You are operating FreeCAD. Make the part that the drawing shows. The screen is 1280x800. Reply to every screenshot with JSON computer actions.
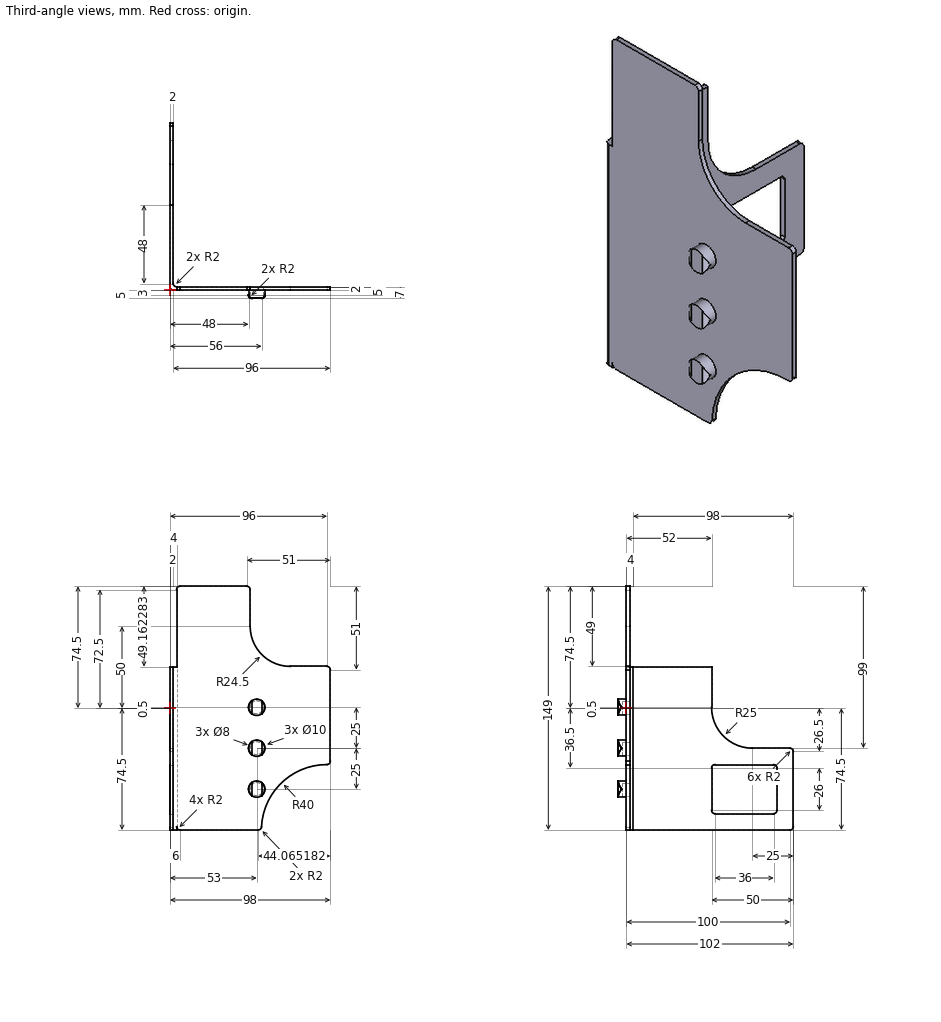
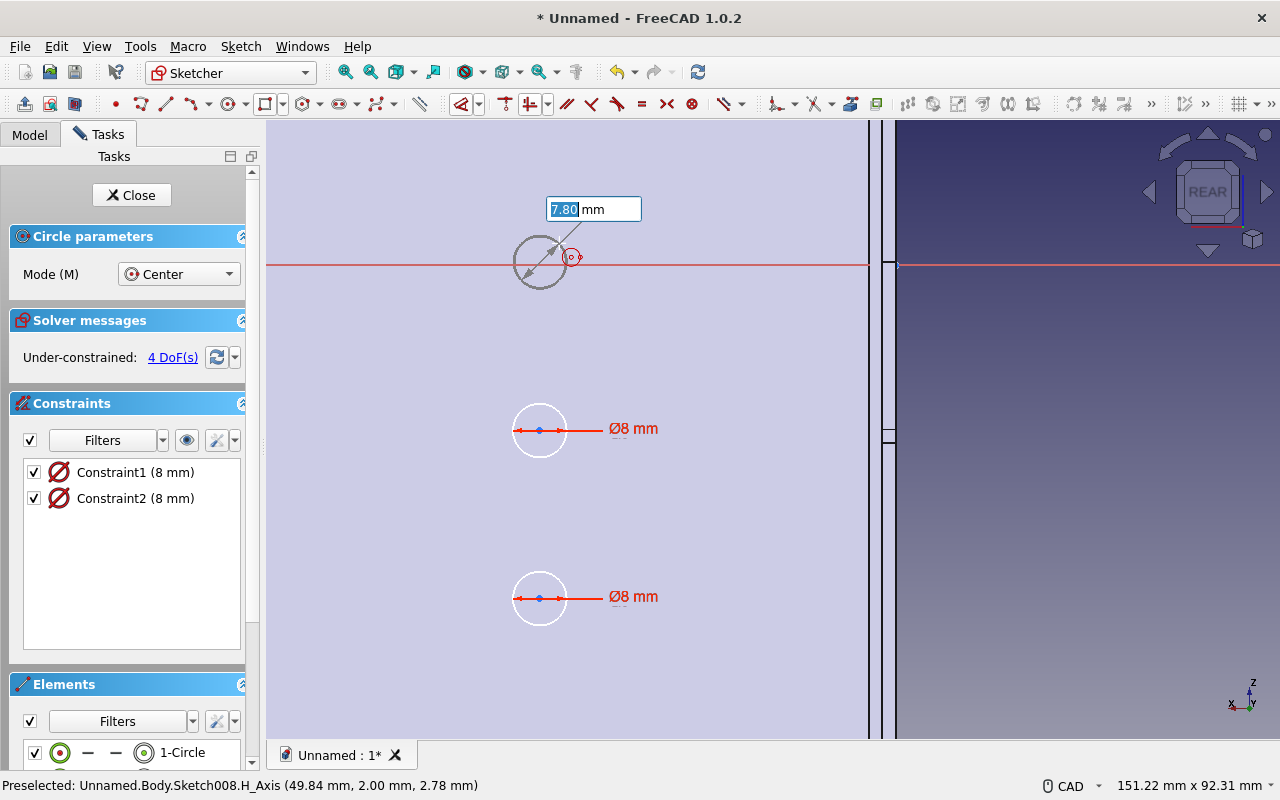
{"action": "type", "text": "8"}
{"action": "key", "text": "Return"}
{"action": "key", "text": "Escape"}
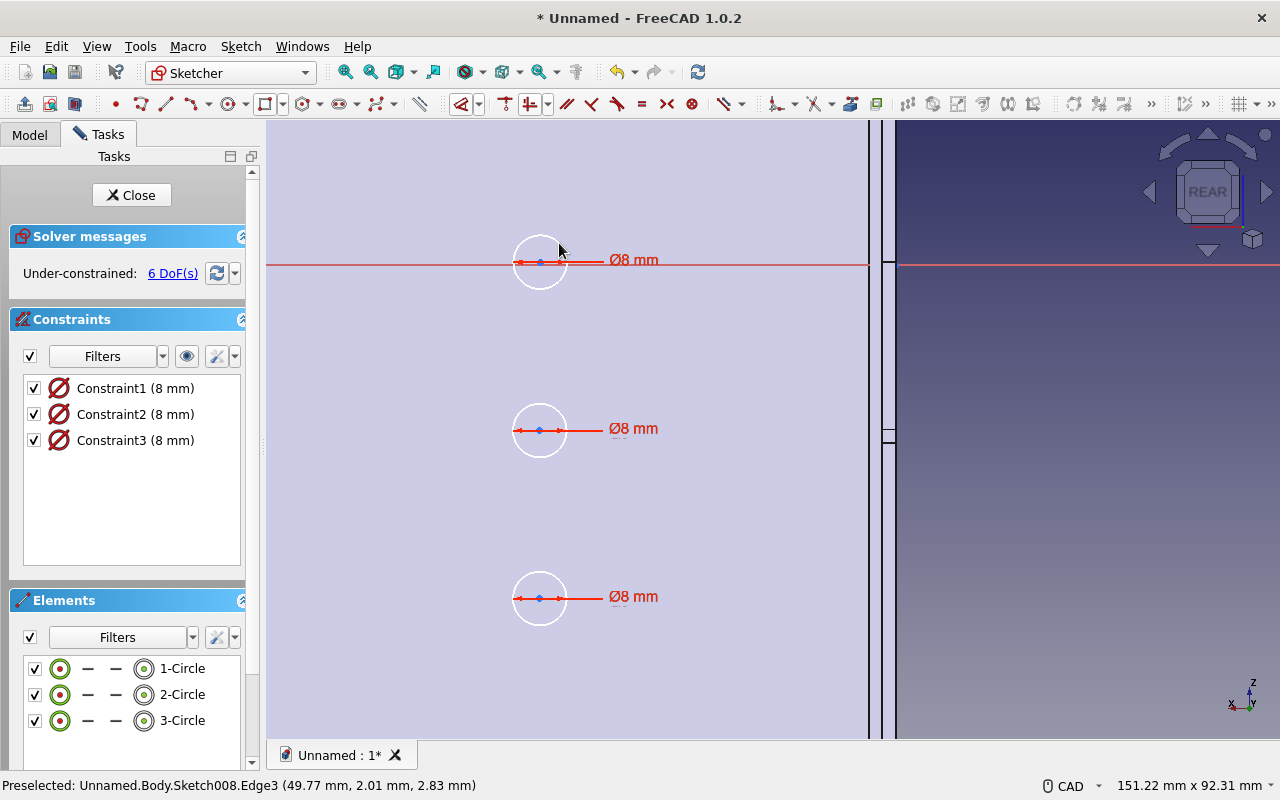
{"action": "left_click", "coordinate": [540, 431]}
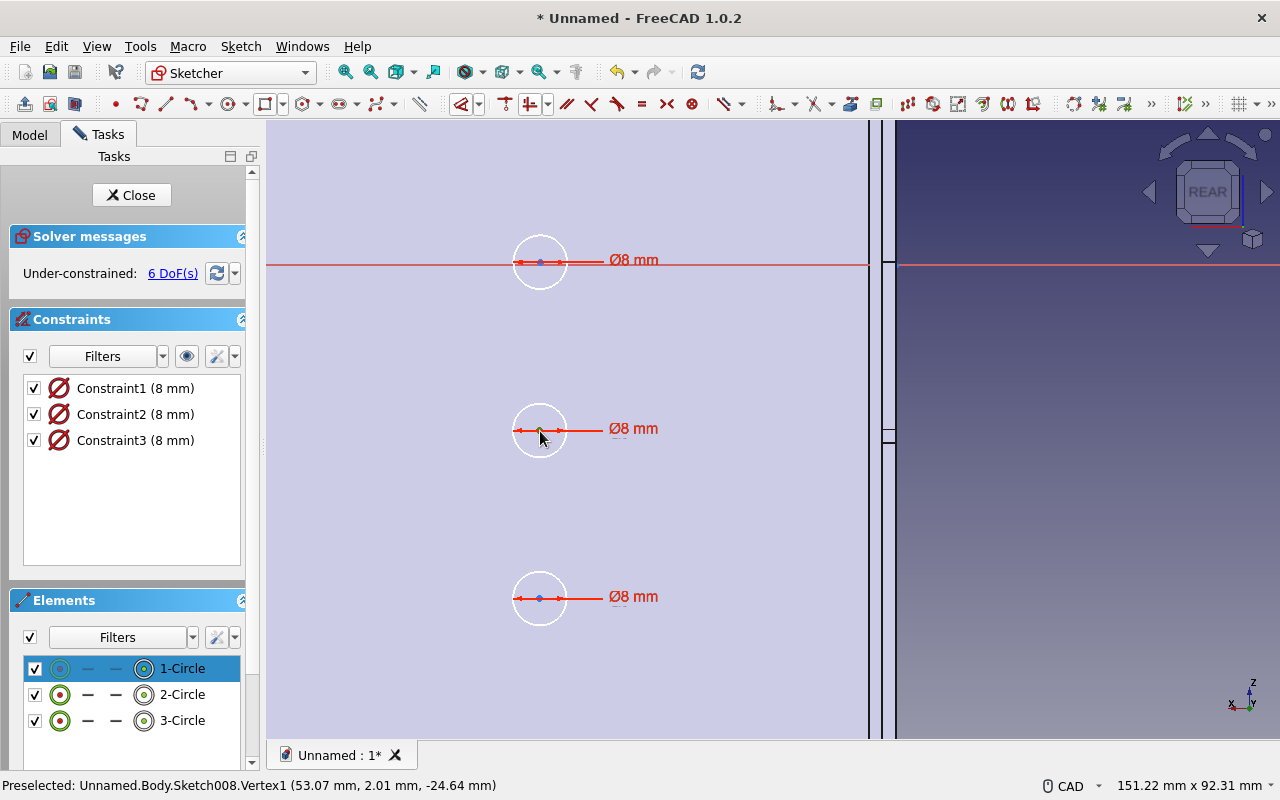
{"action": "left_click", "coordinate": [540, 599]}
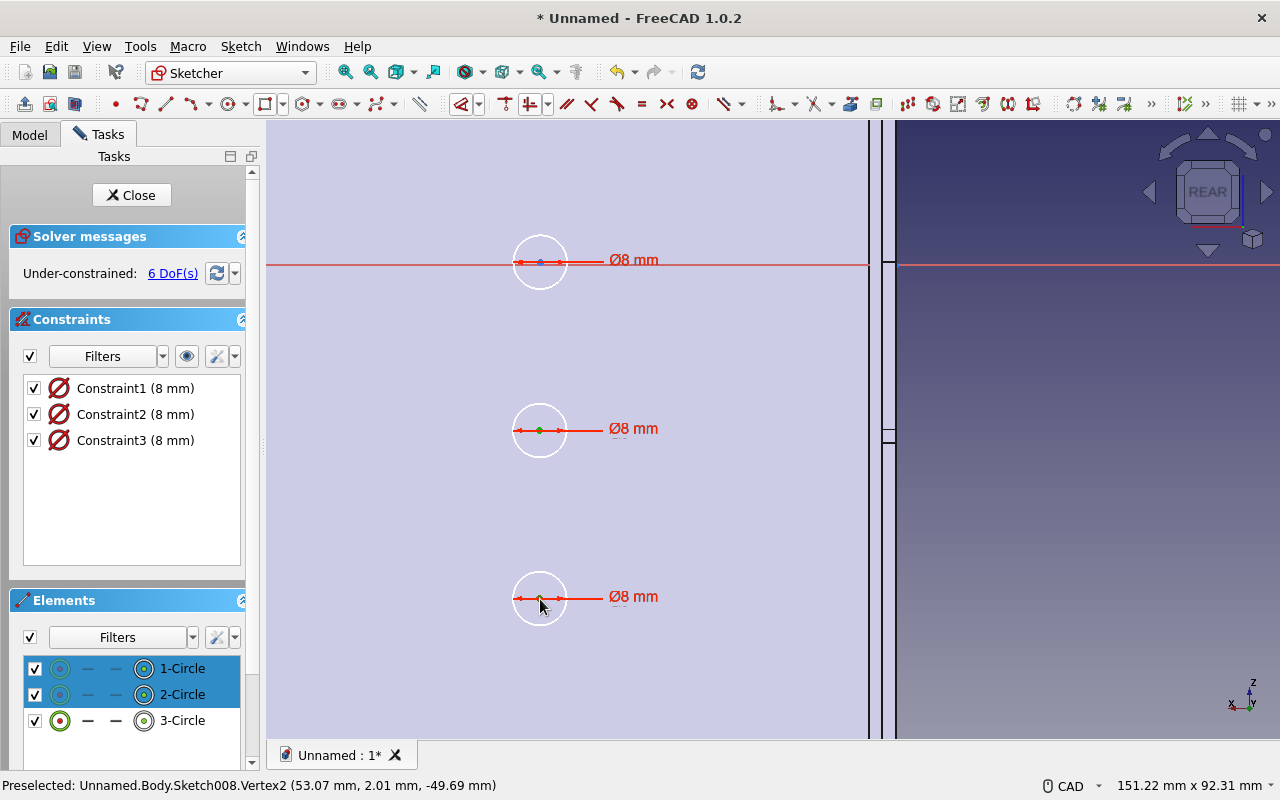
{"action": "key", "text": "v"}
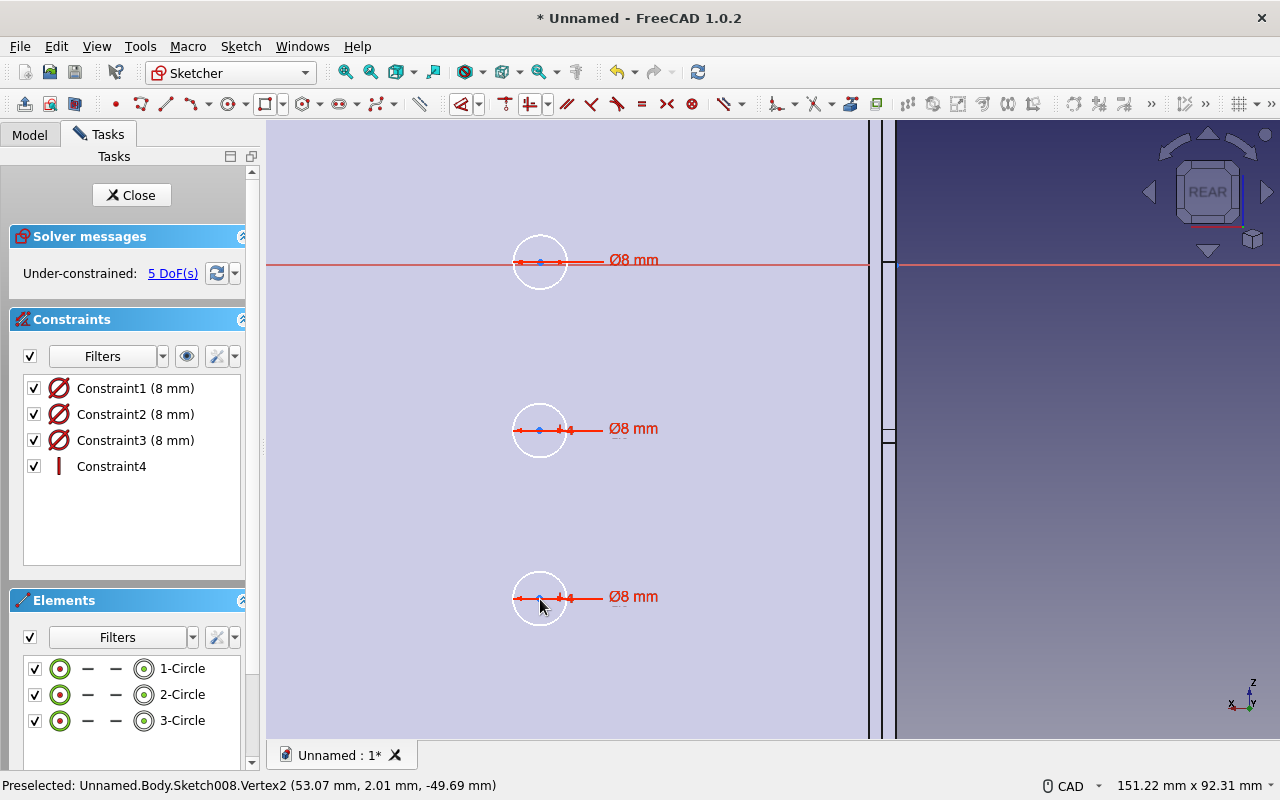
{"action": "left_click", "coordinate": [540, 431]}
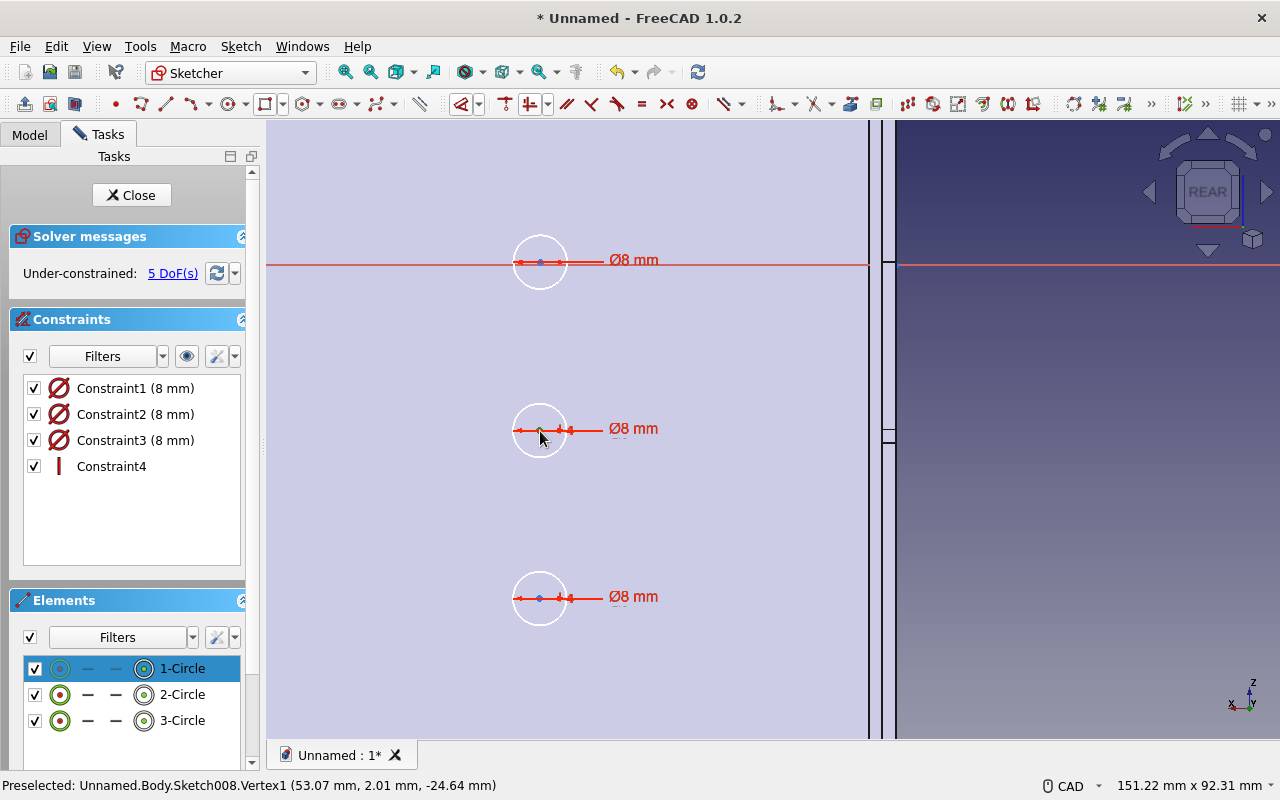
{"action": "left_click", "coordinate": [540, 262]}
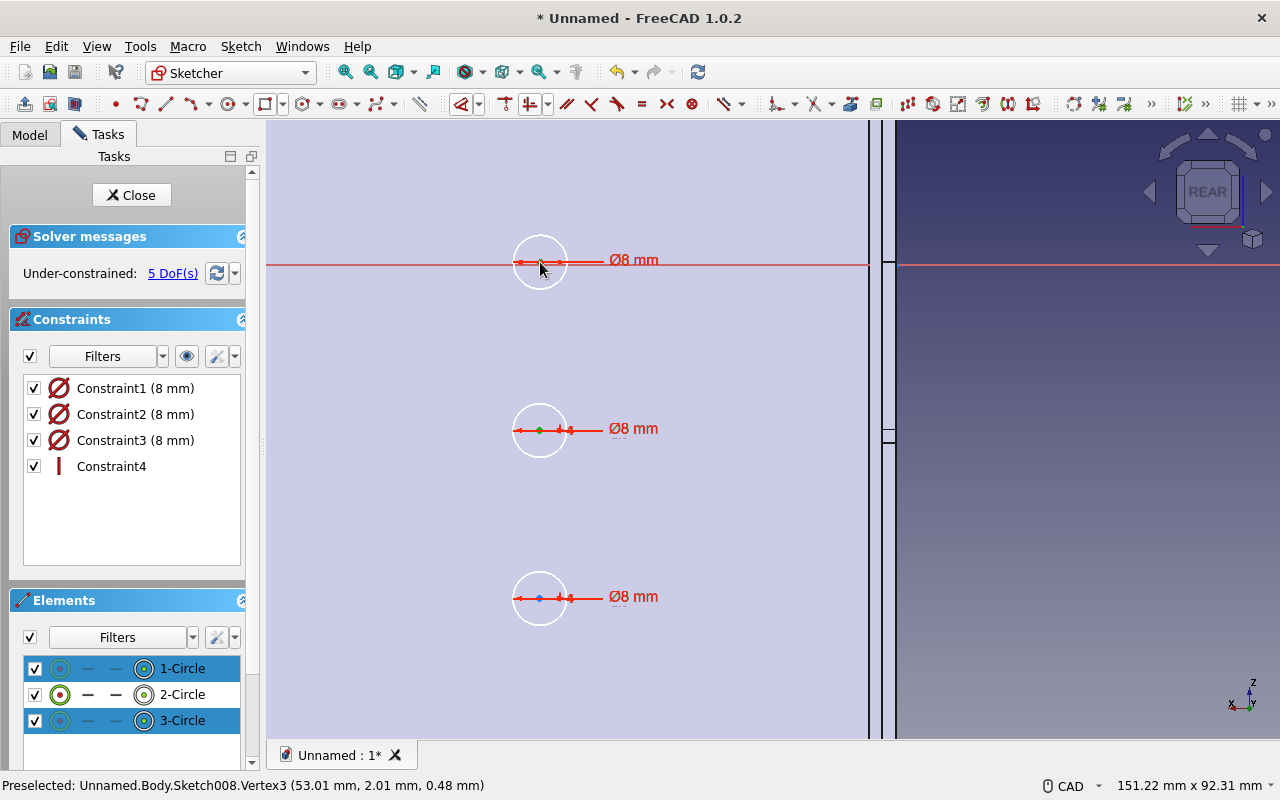
{"action": "key", "text": "v"}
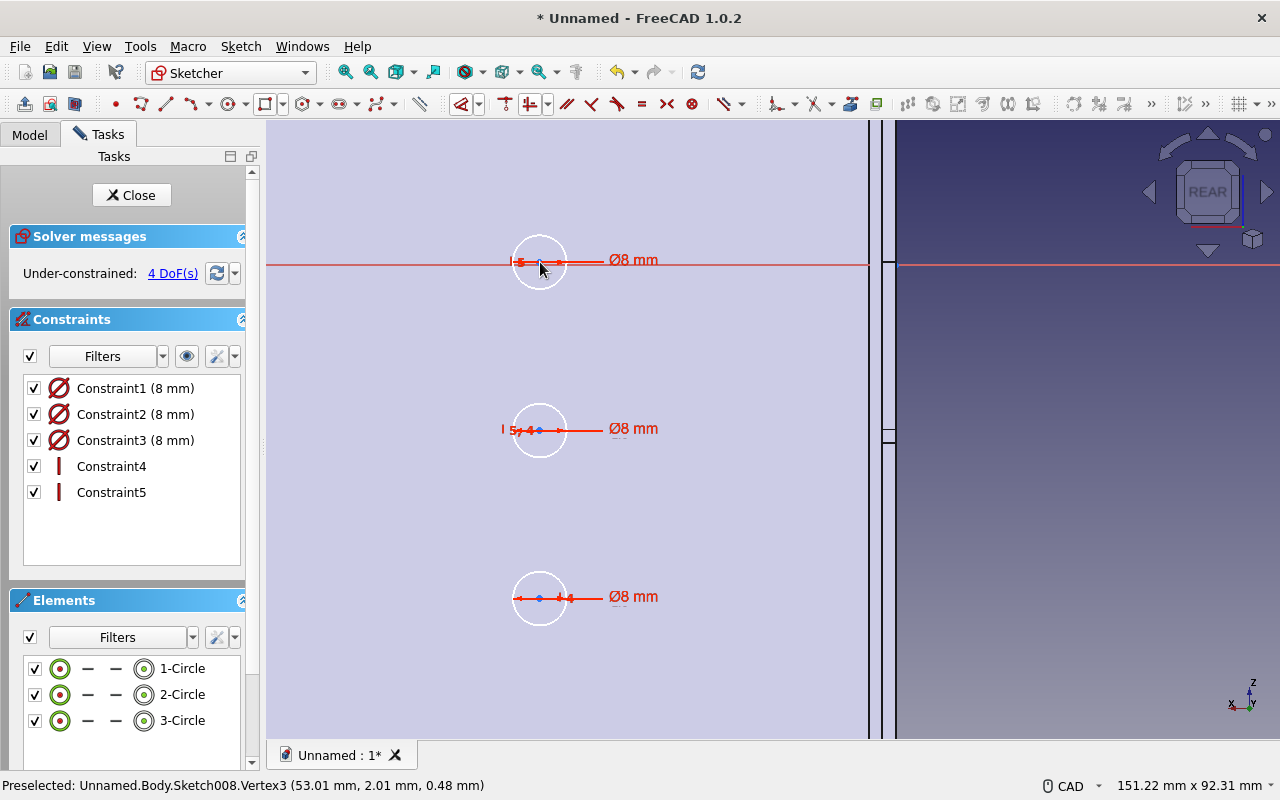
{"action": "left_click", "coordinate": [540, 431]}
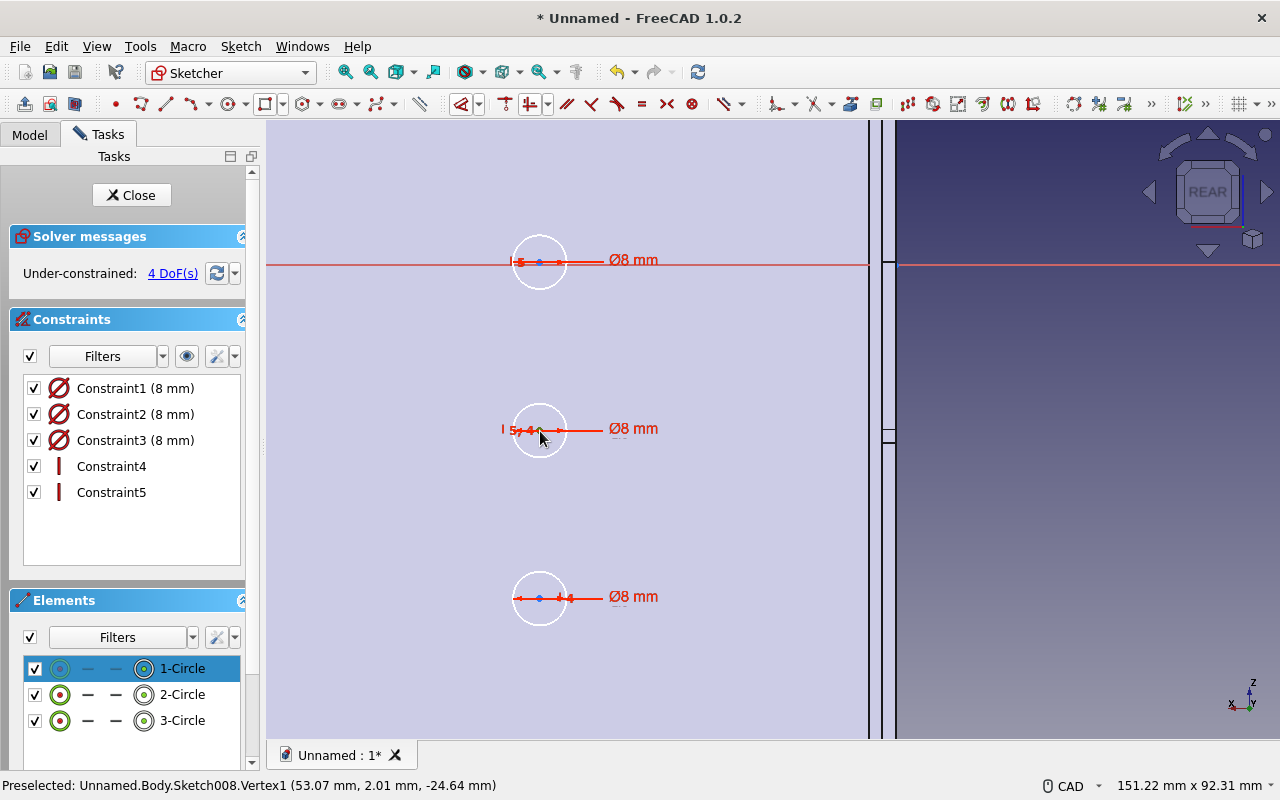
{"action": "key", "text": "l"}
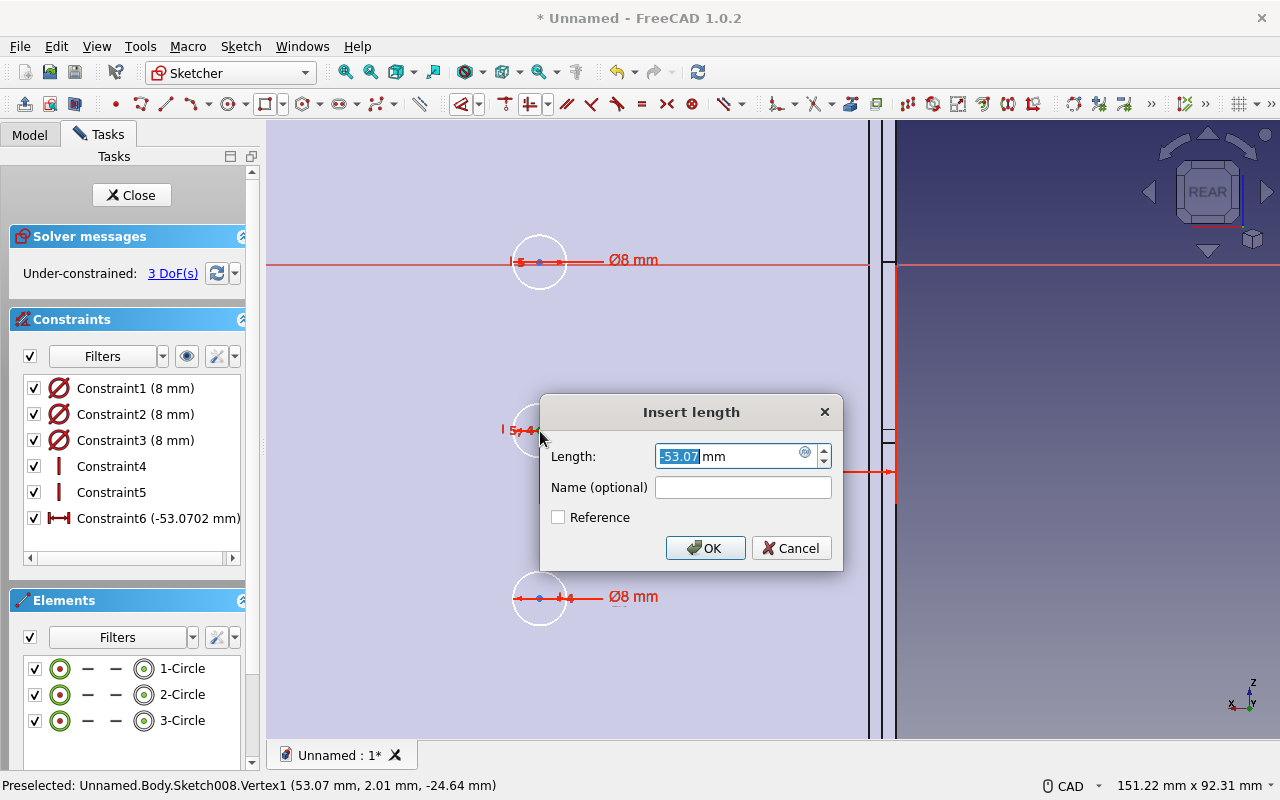
{"action": "type", "text": "-53"}
{"action": "key", "text": "Return"}